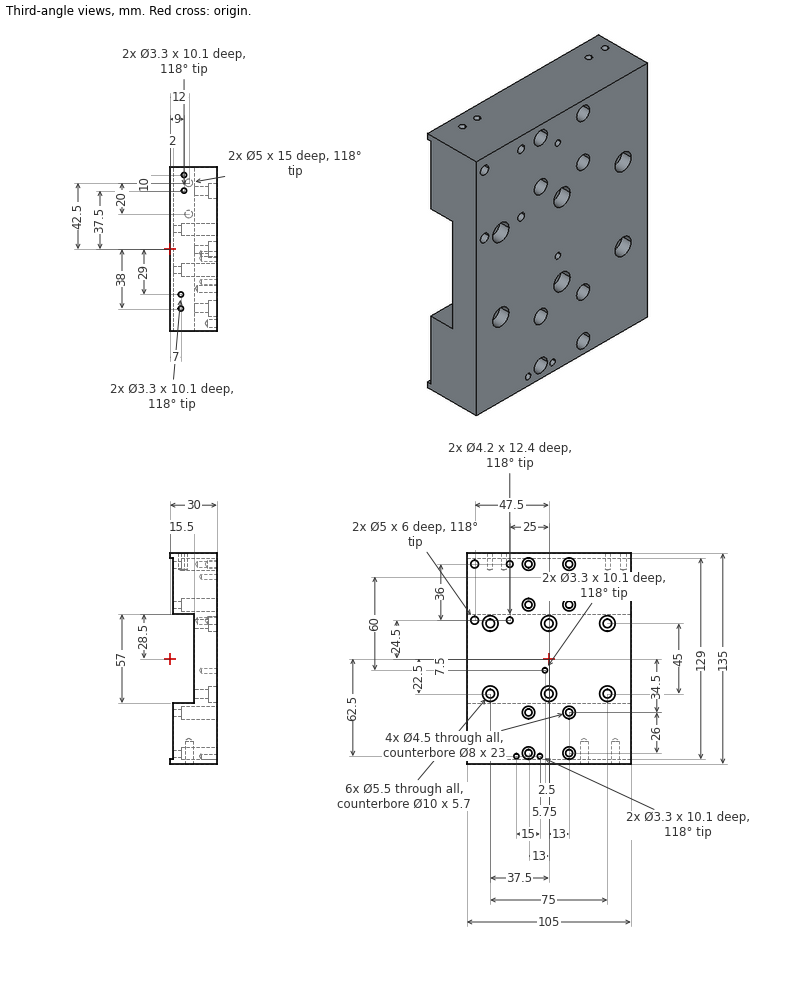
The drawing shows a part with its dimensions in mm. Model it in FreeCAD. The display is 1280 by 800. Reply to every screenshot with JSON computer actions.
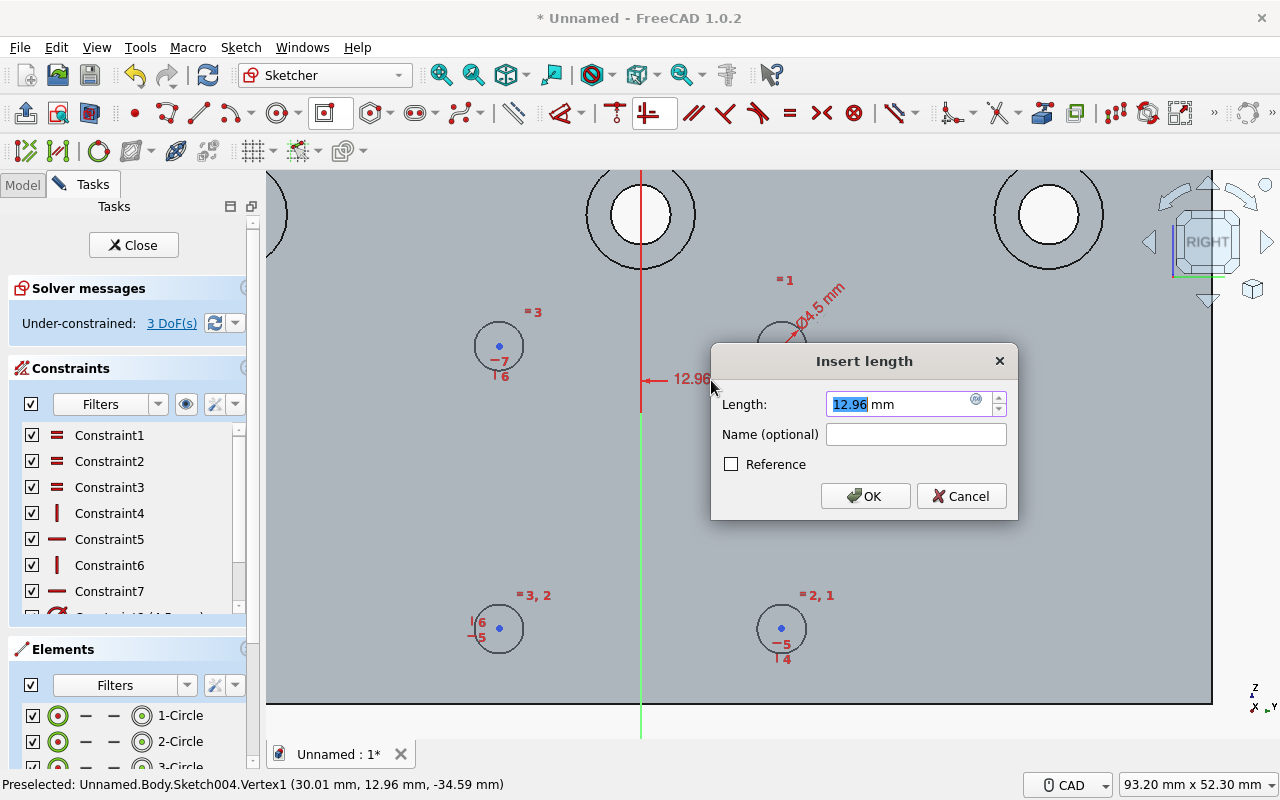
{"action": "type", "text": "13"}
{"action": "key", "text": "Return"}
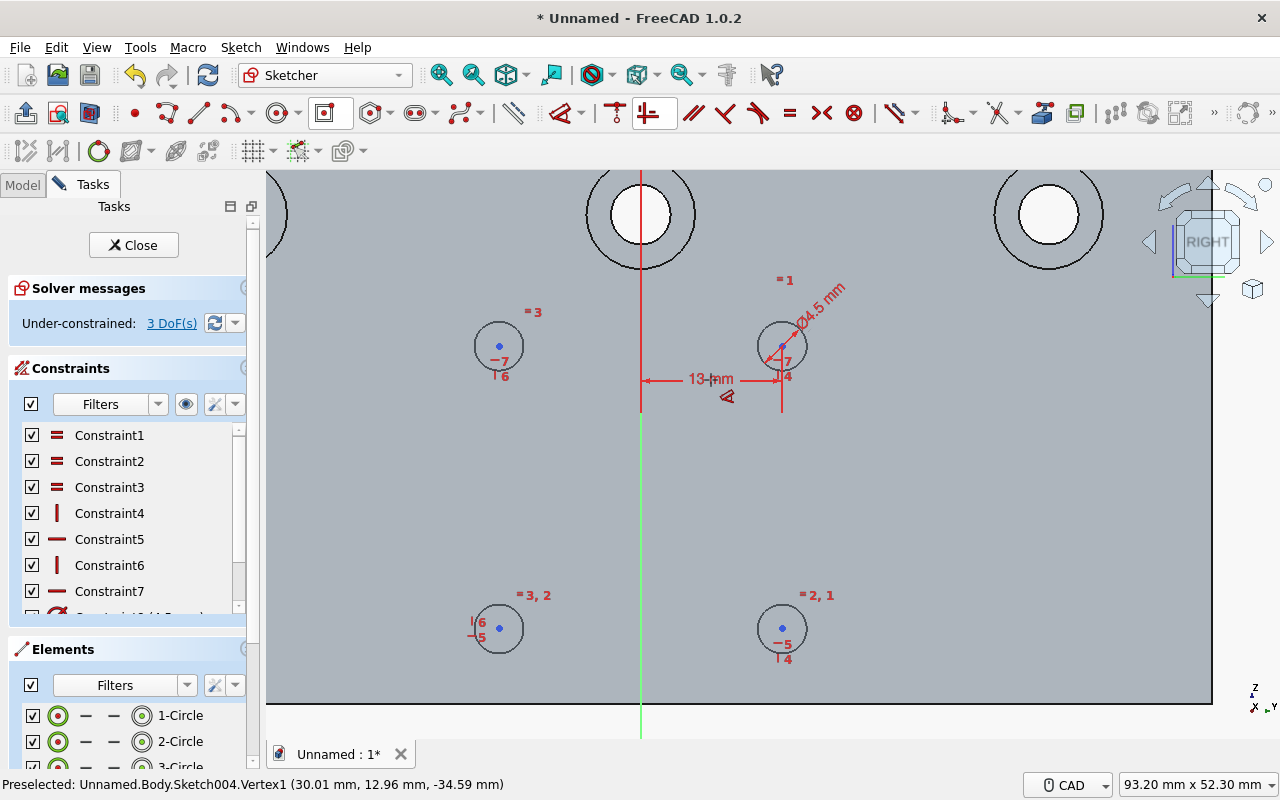
{"action": "left_click", "coordinate": [499, 629]}
{"action": "left_click", "coordinate": [570, 663]}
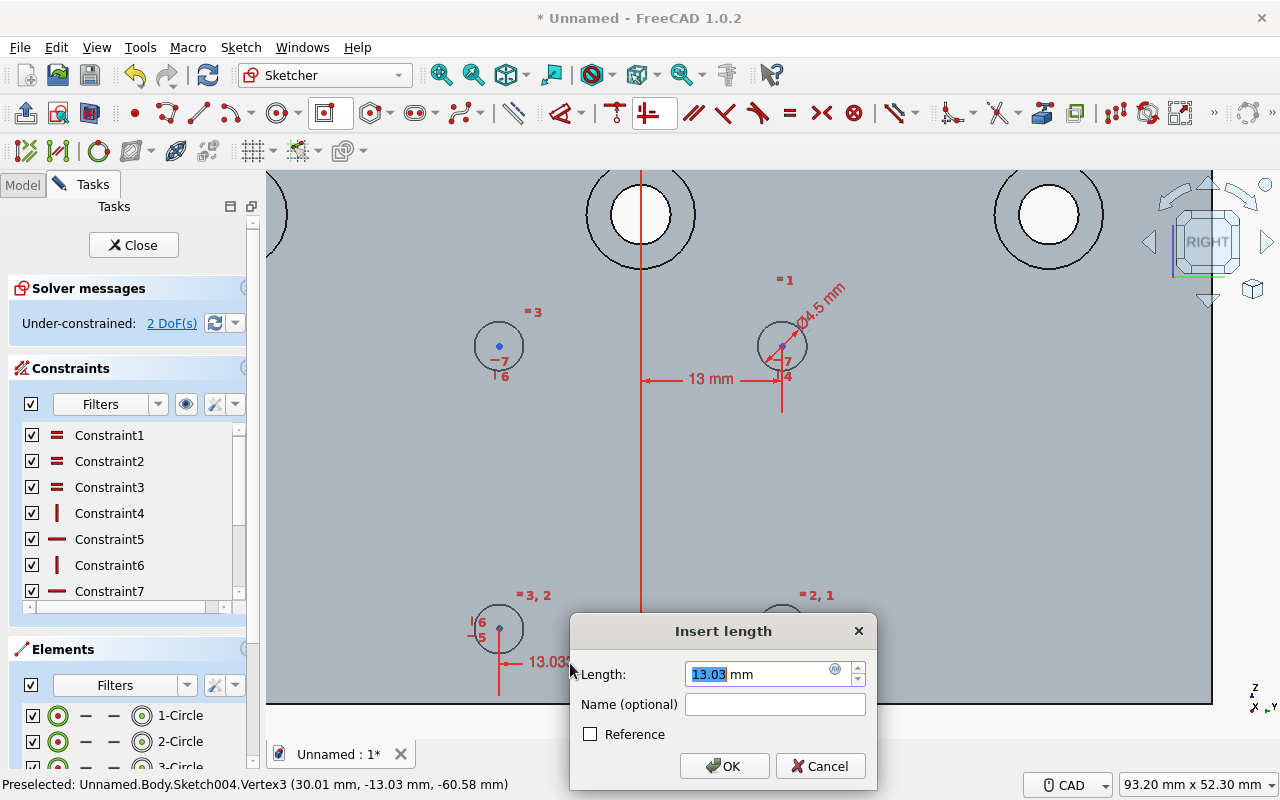
{"action": "type", "text": "13"}
{"action": "key", "text": "Return"}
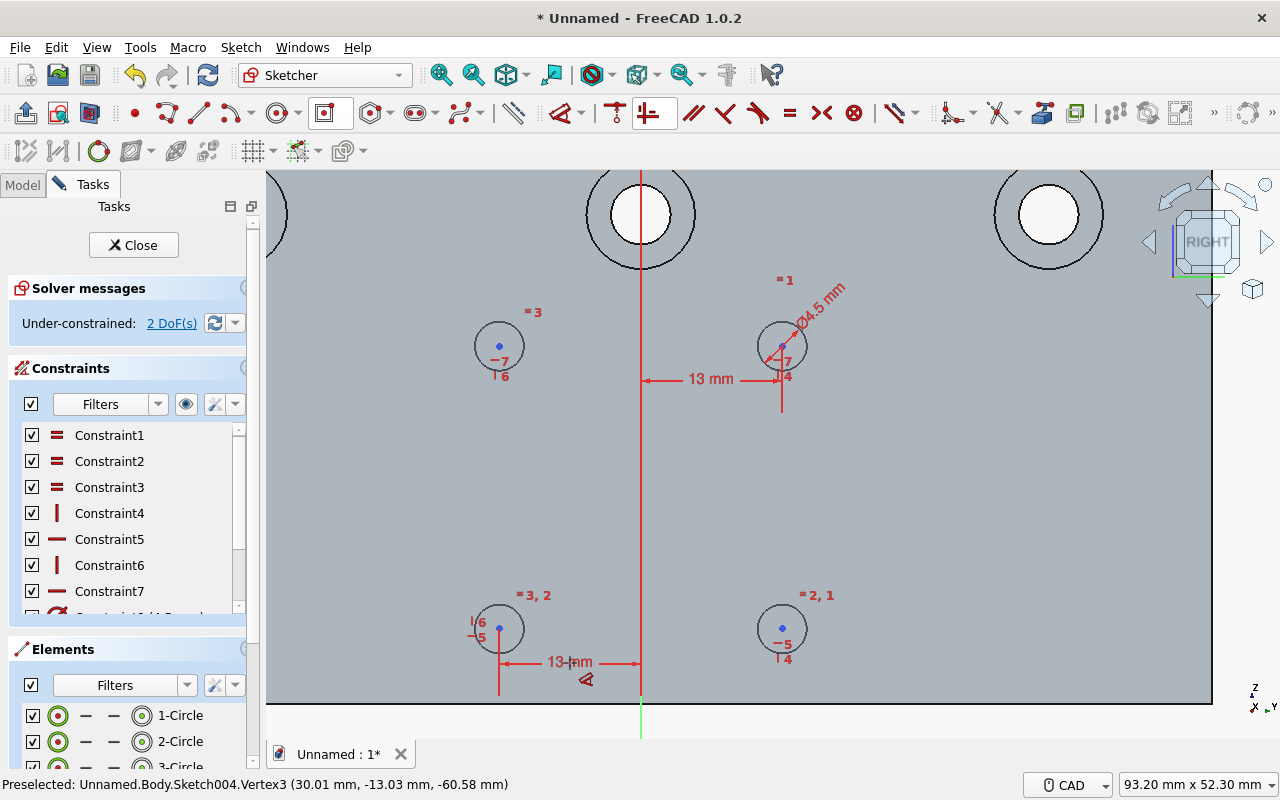
{"action": "left_click", "coordinate": [782, 346]}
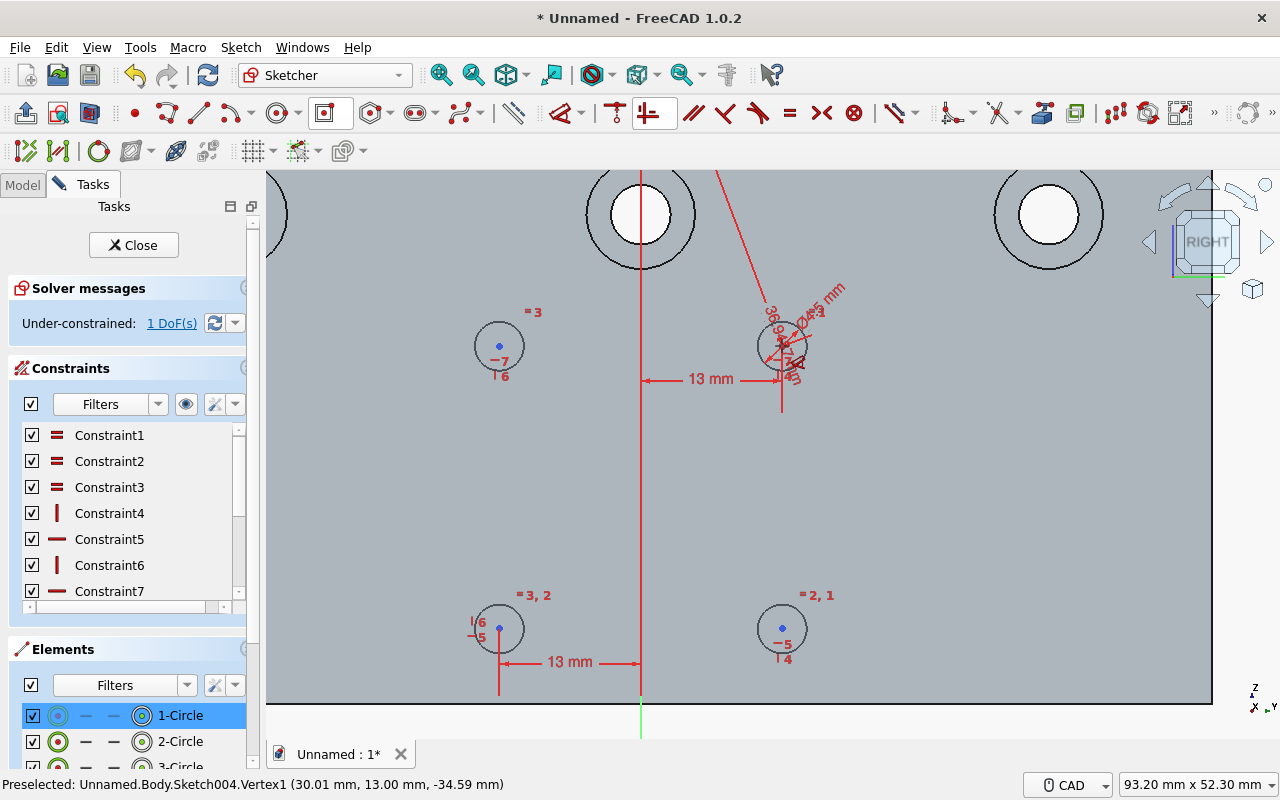
{"action": "left_click", "coordinate": [782, 629]}
{"action": "left_click", "coordinate": [816, 488]}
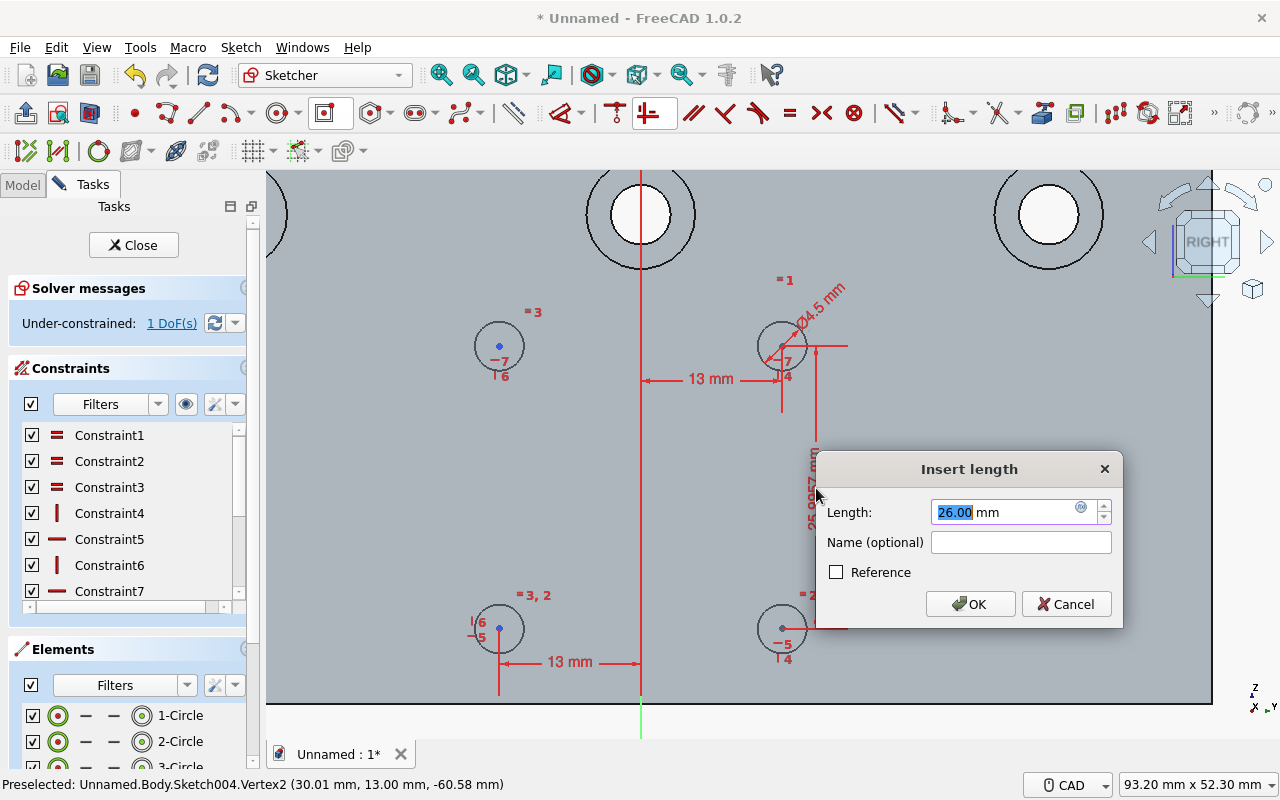
{"action": "type", "text": "26"}
{"action": "key", "text": "Return"}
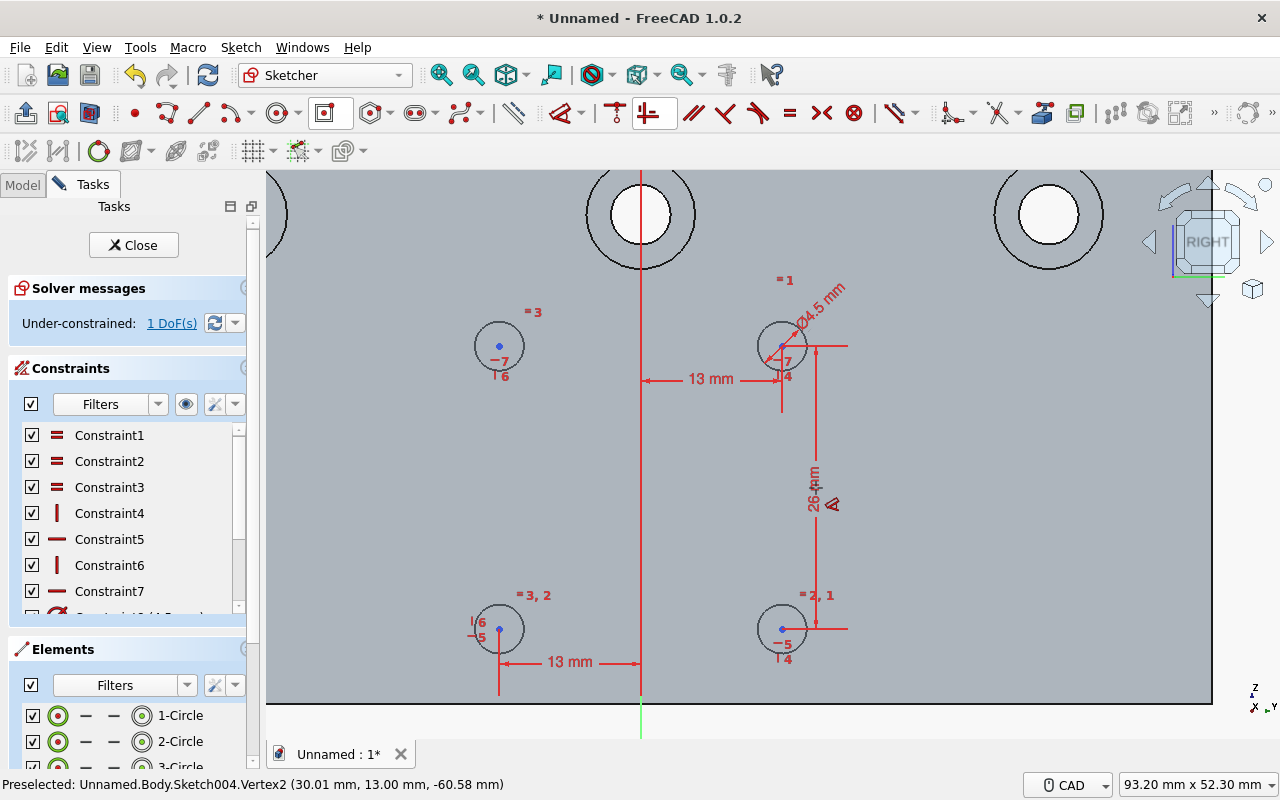
{"action": "left_click", "coordinate": [782, 346]}
{"action": "left_click", "coordinate": [816, 272]}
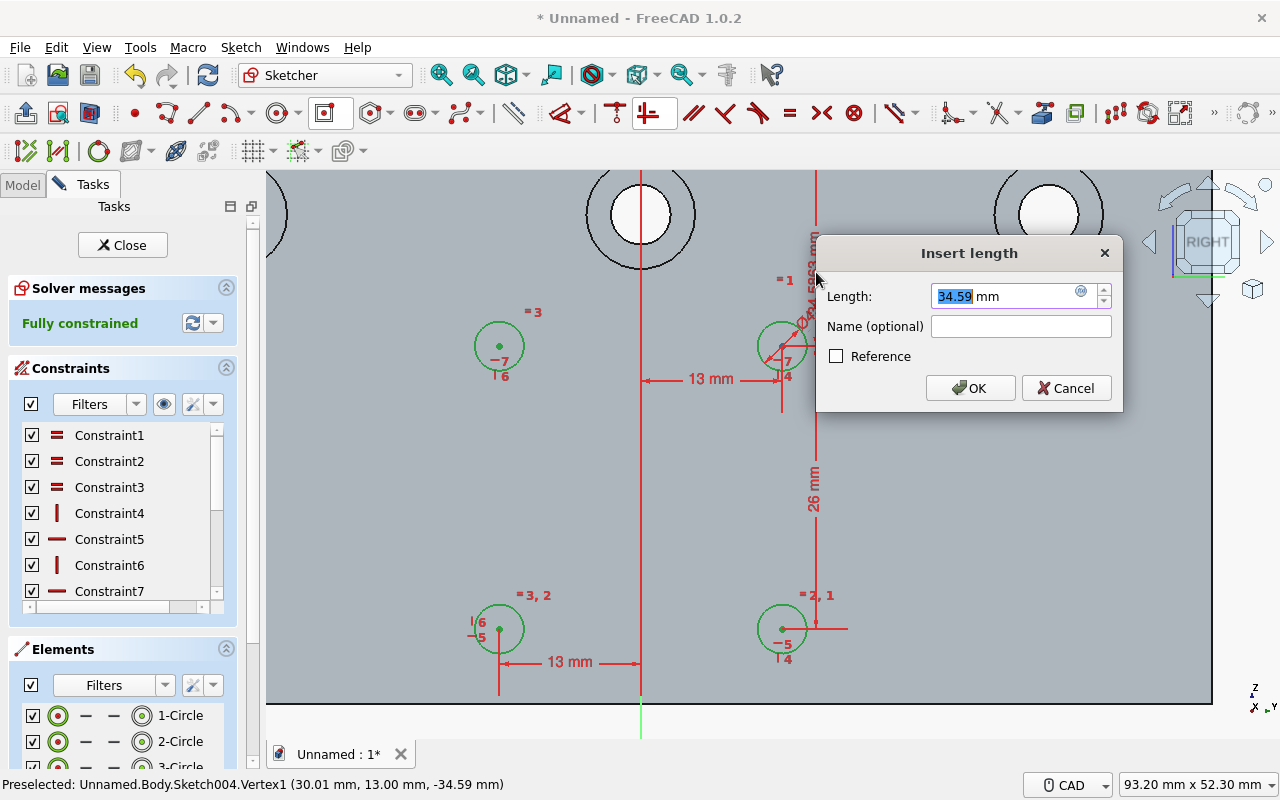
{"action": "type", "text": "34.5"}
{"action": "key", "text": "Return"}
{"action": "key", "text": "Escape"}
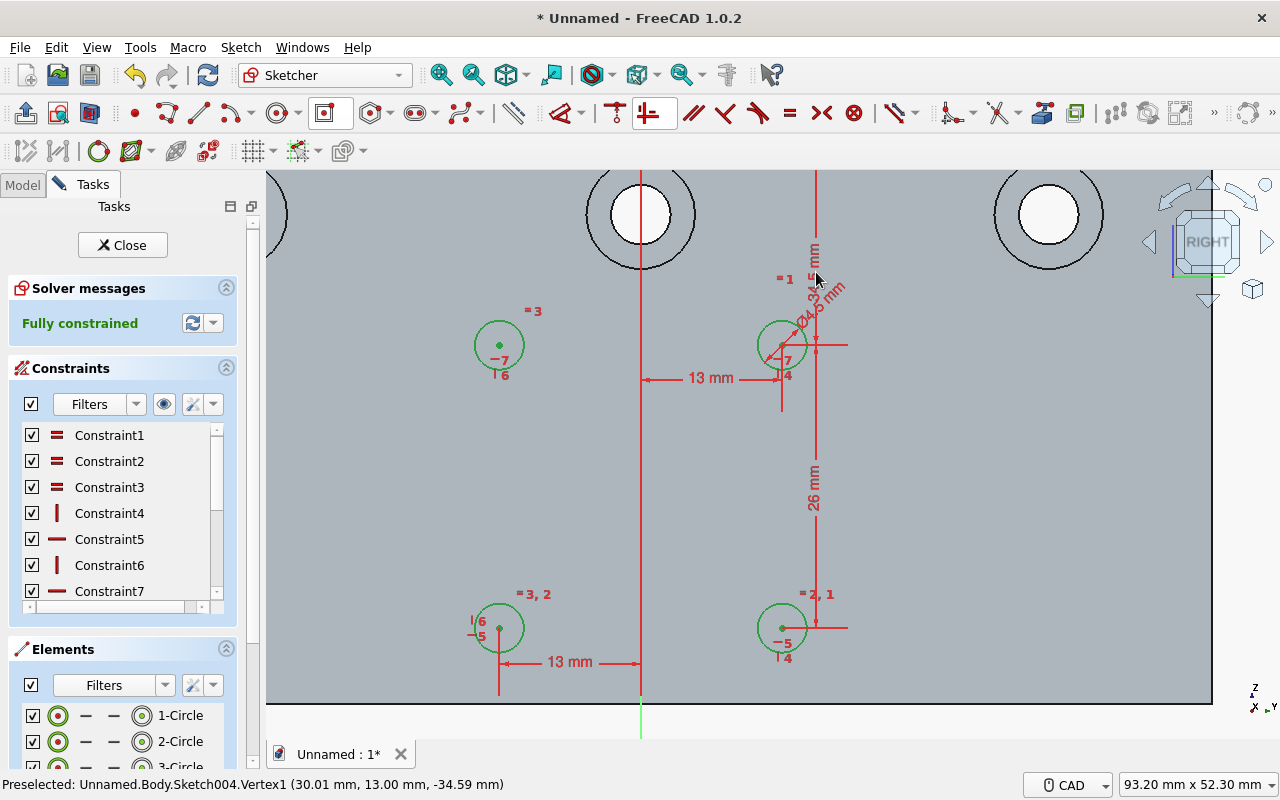
{"action": "left_click", "coordinate": [123, 245]}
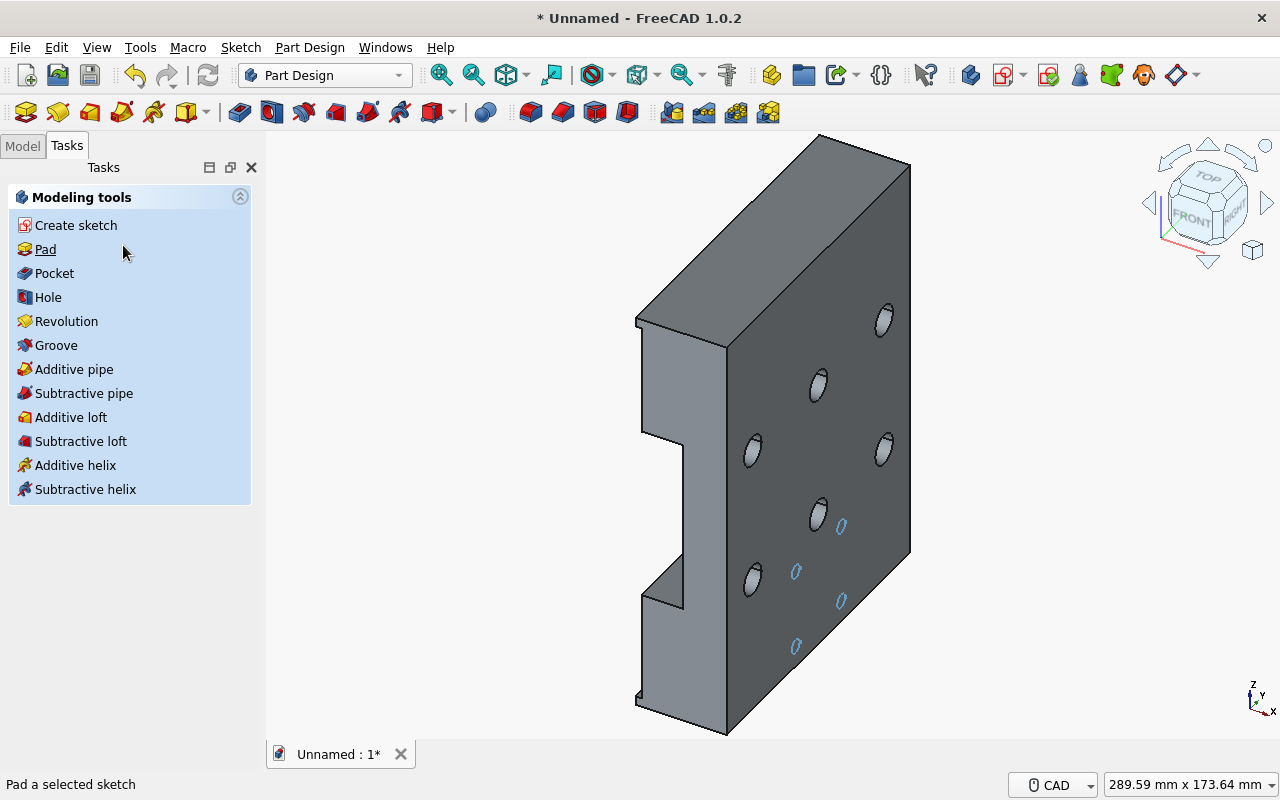
{"action": "left_click", "coordinate": [272, 112]}